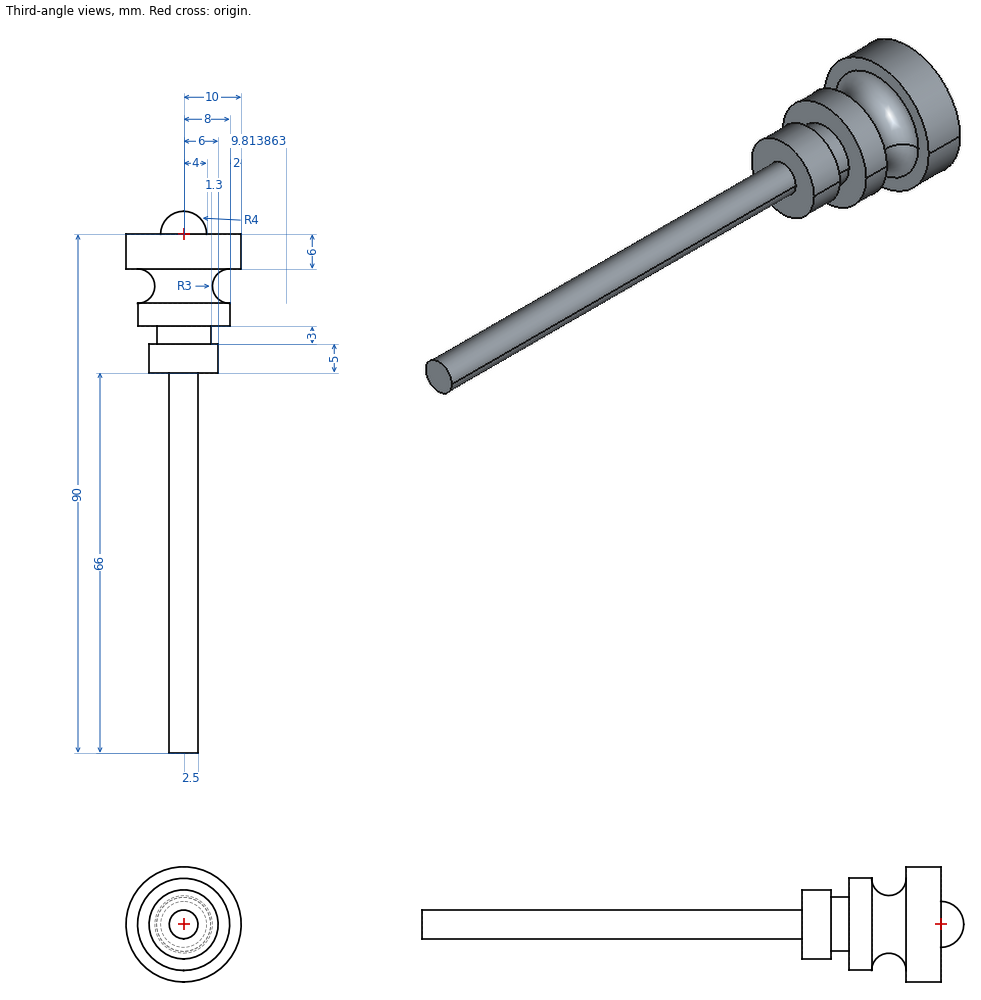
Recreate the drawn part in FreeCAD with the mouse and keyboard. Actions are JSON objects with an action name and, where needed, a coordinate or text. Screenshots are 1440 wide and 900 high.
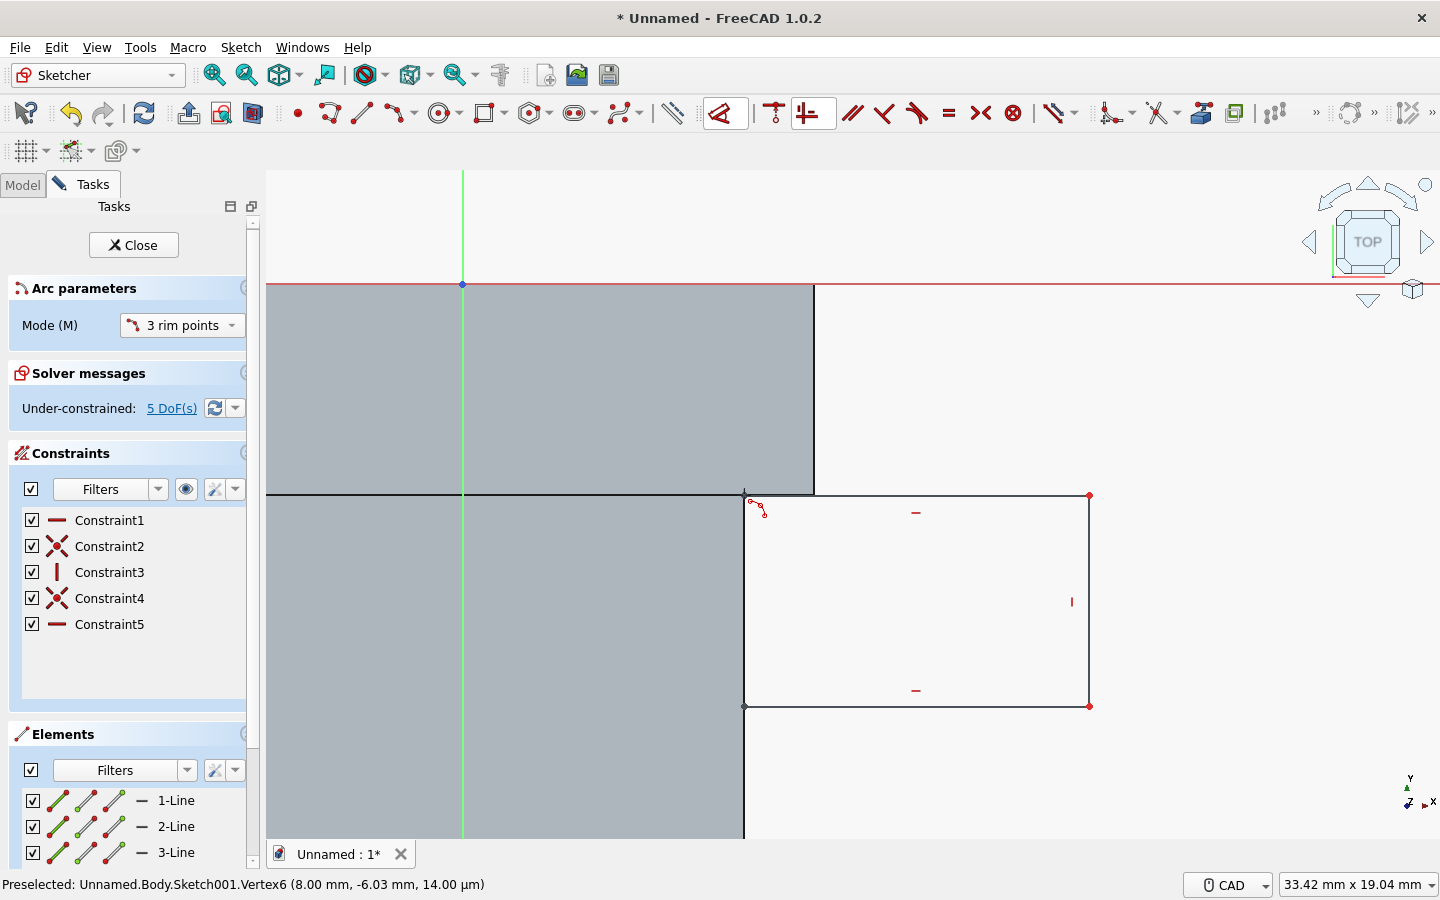
{"action": "left_click", "coordinate": [744, 496]}
{"action": "left_click", "coordinate": [744, 707]}
{"action": "left_click", "coordinate": [639, 600]}
{"action": "key", "text": "Escape"}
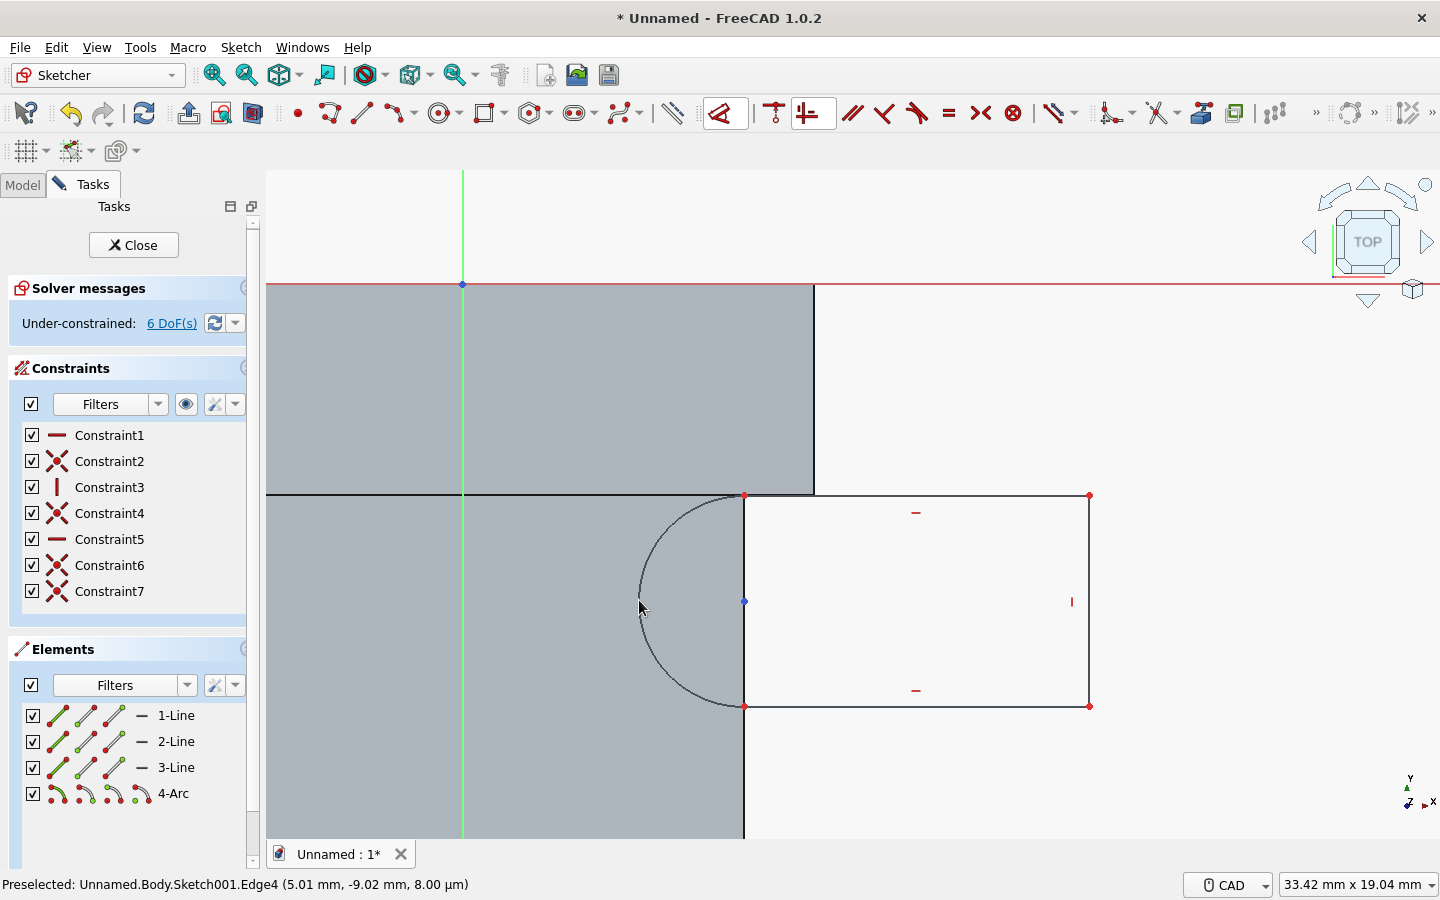
{"action": "left_click", "coordinate": [847, 707]}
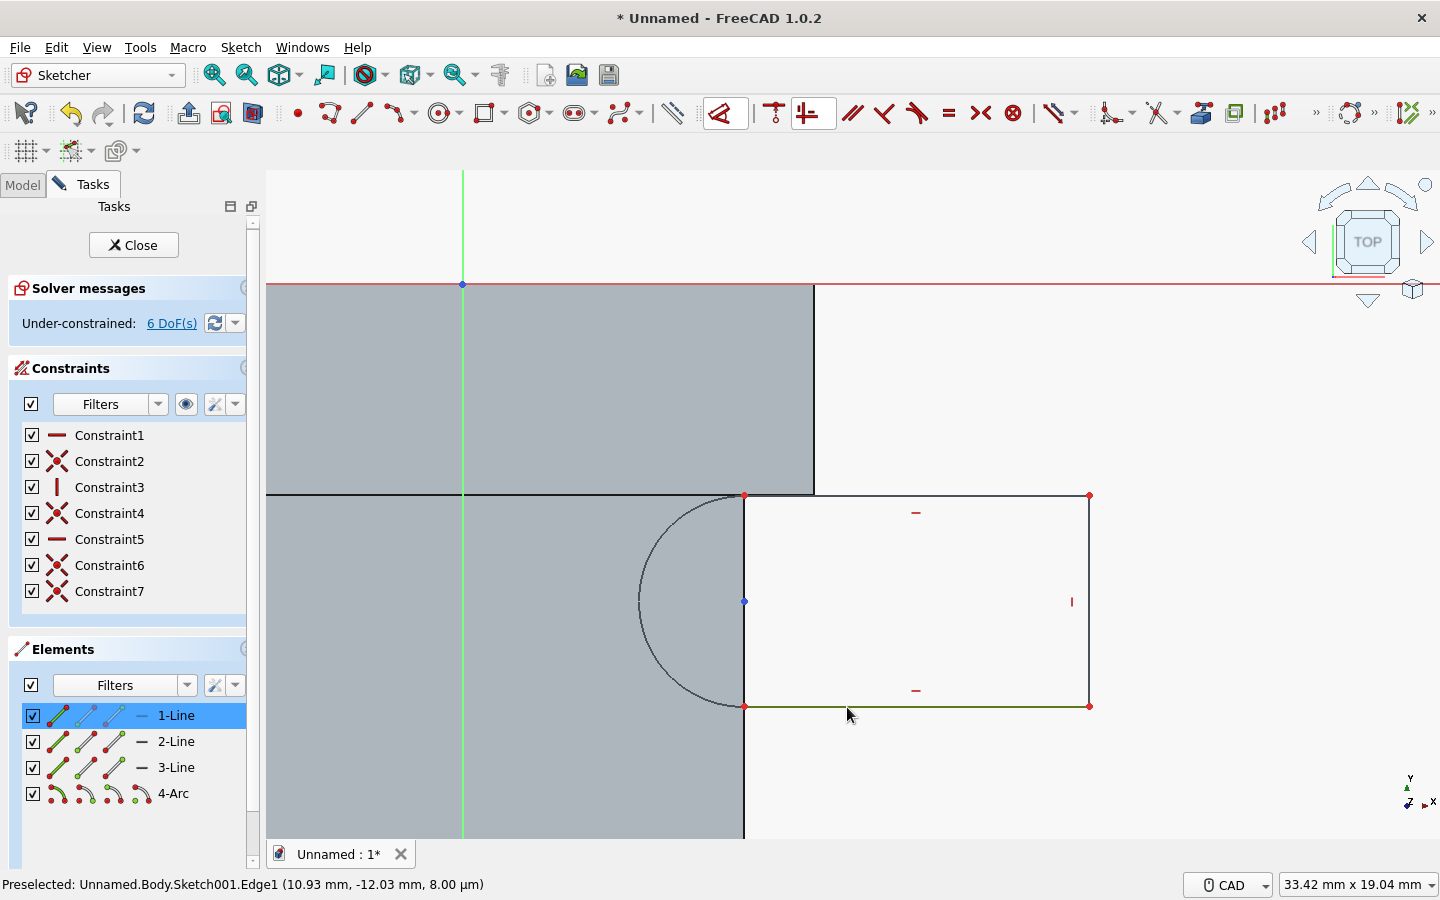
{"action": "left_click", "coordinate": [659, 540]}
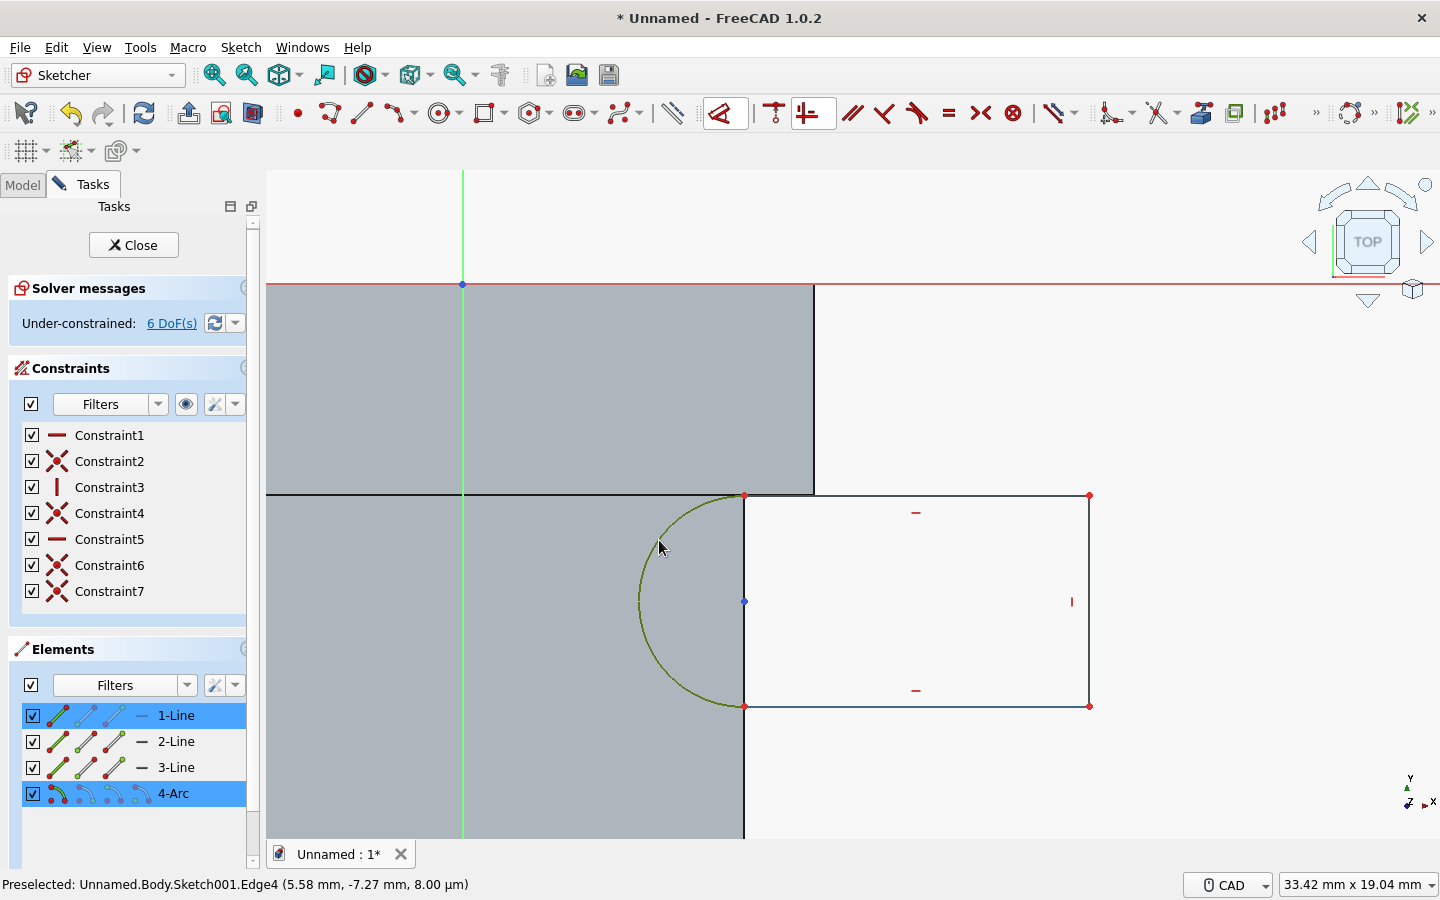
{"action": "key", "text": "t"}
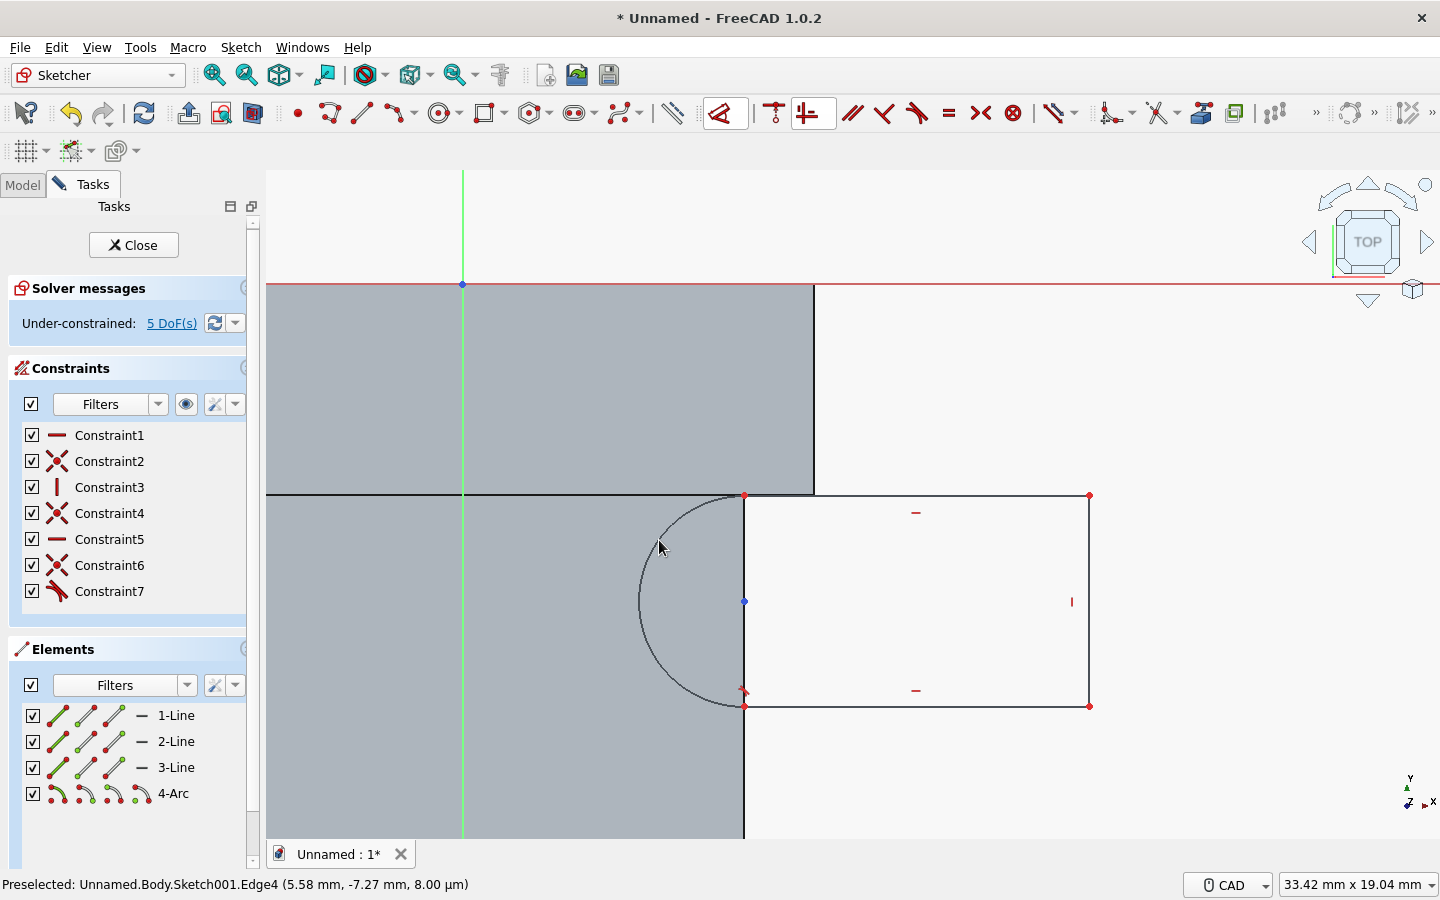
{"action": "left_click", "coordinate": [986, 496]}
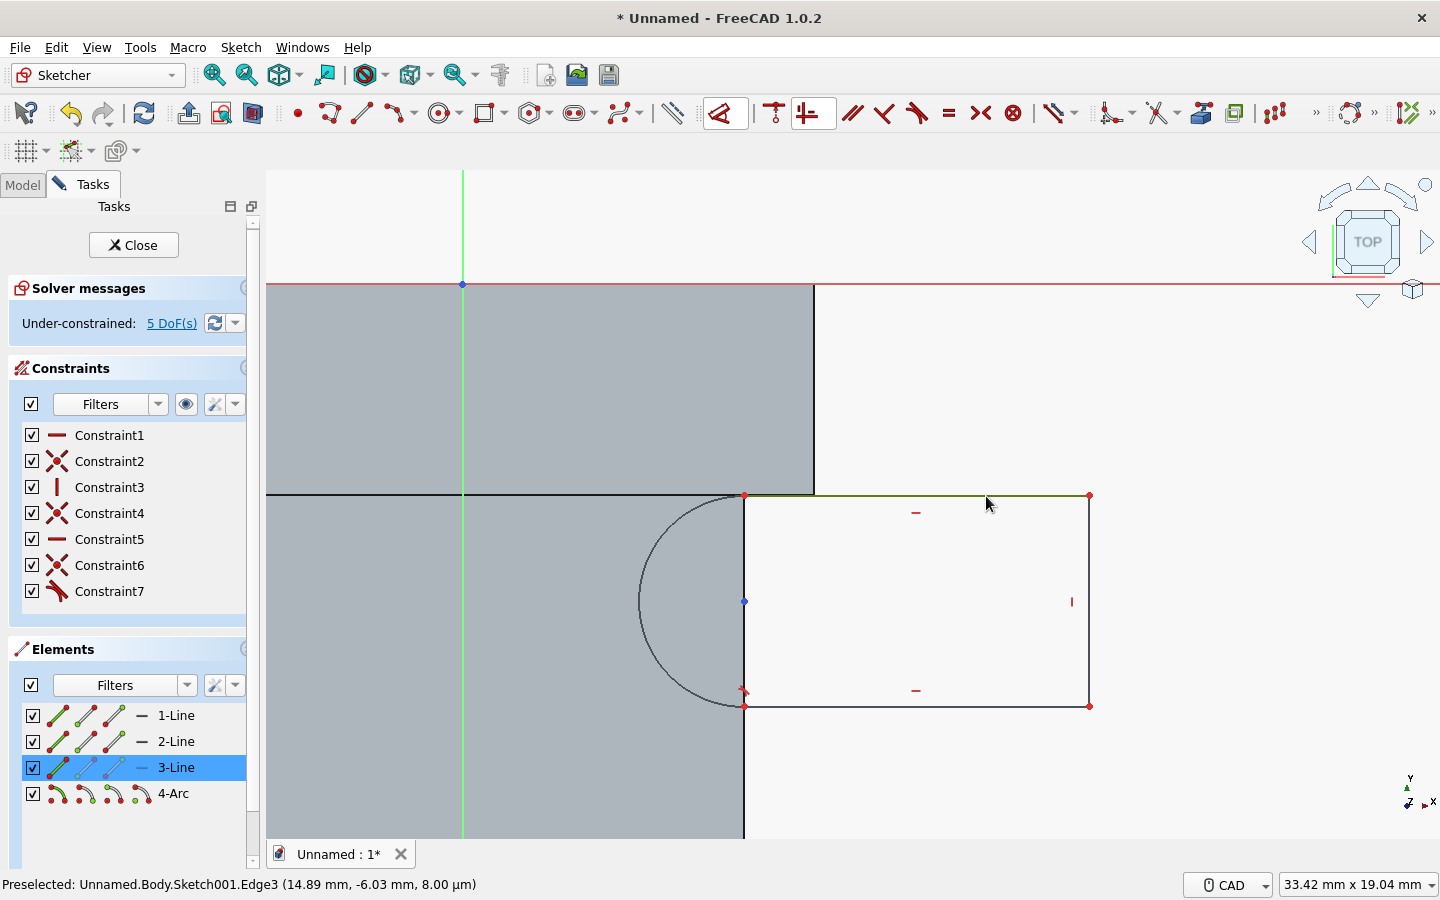
{"action": "left_click", "coordinate": [659, 540]}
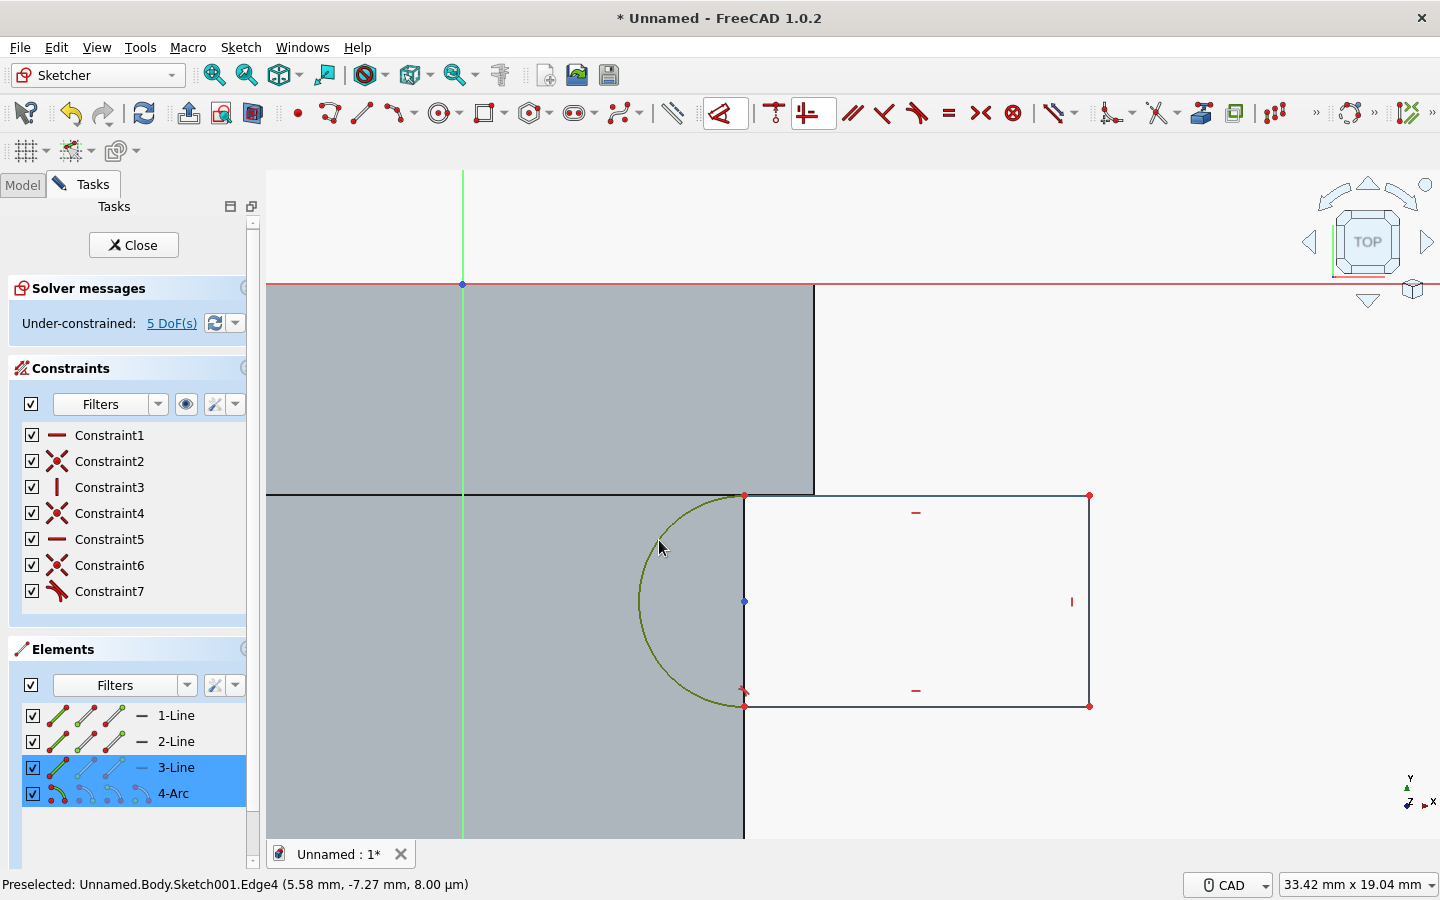
{"action": "left_click", "coordinate": [918, 114]}